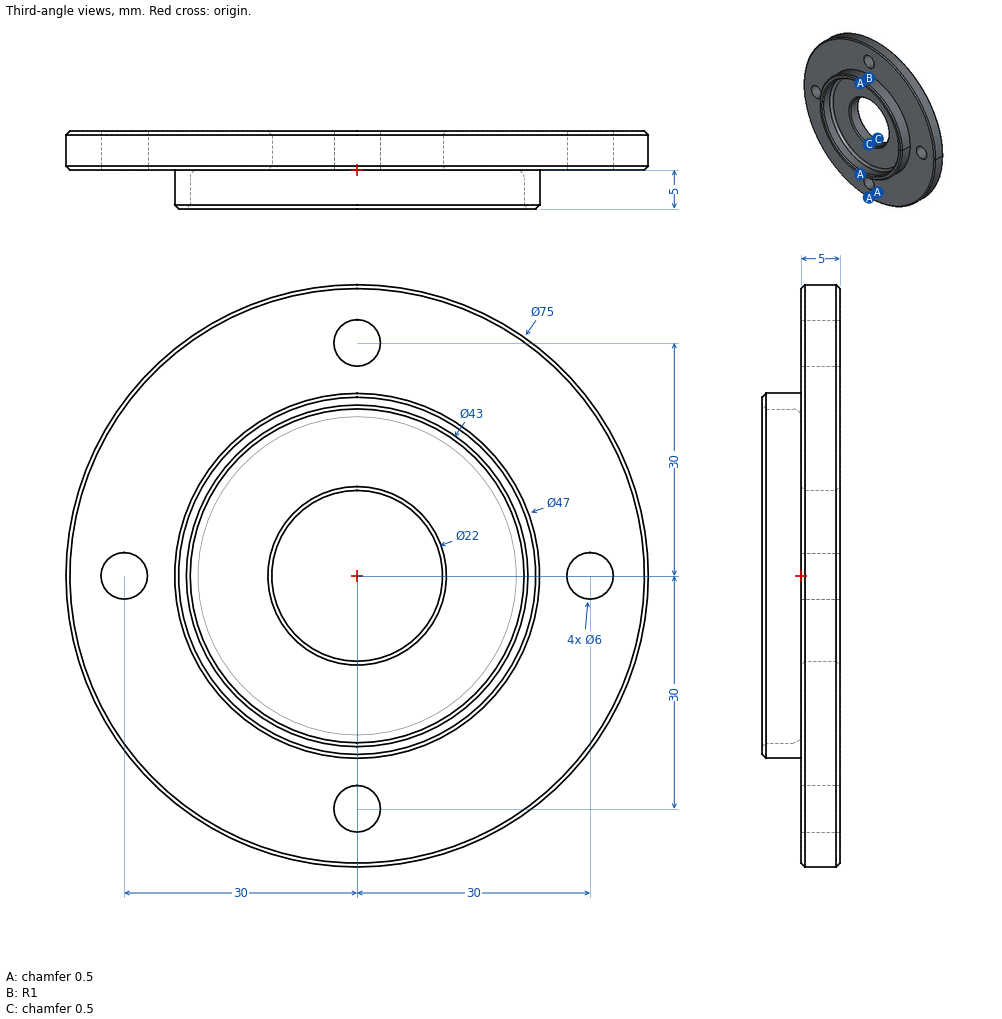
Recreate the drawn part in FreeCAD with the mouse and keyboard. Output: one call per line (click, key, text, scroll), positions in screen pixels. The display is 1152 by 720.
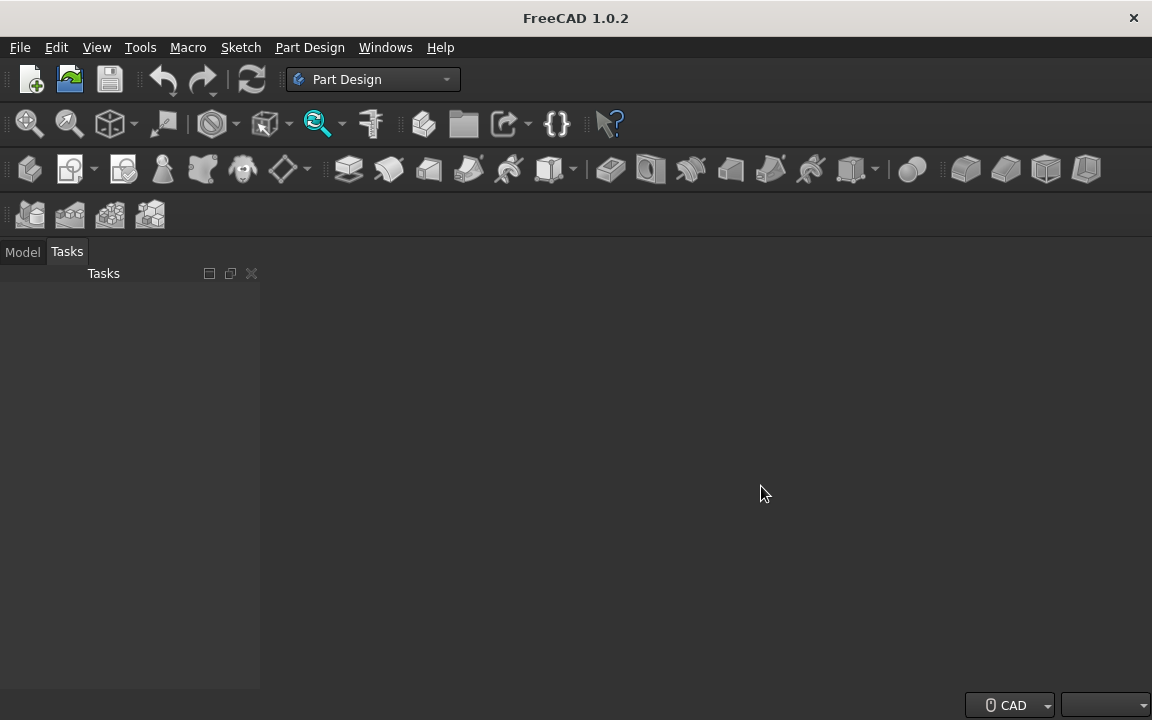
click(30, 80)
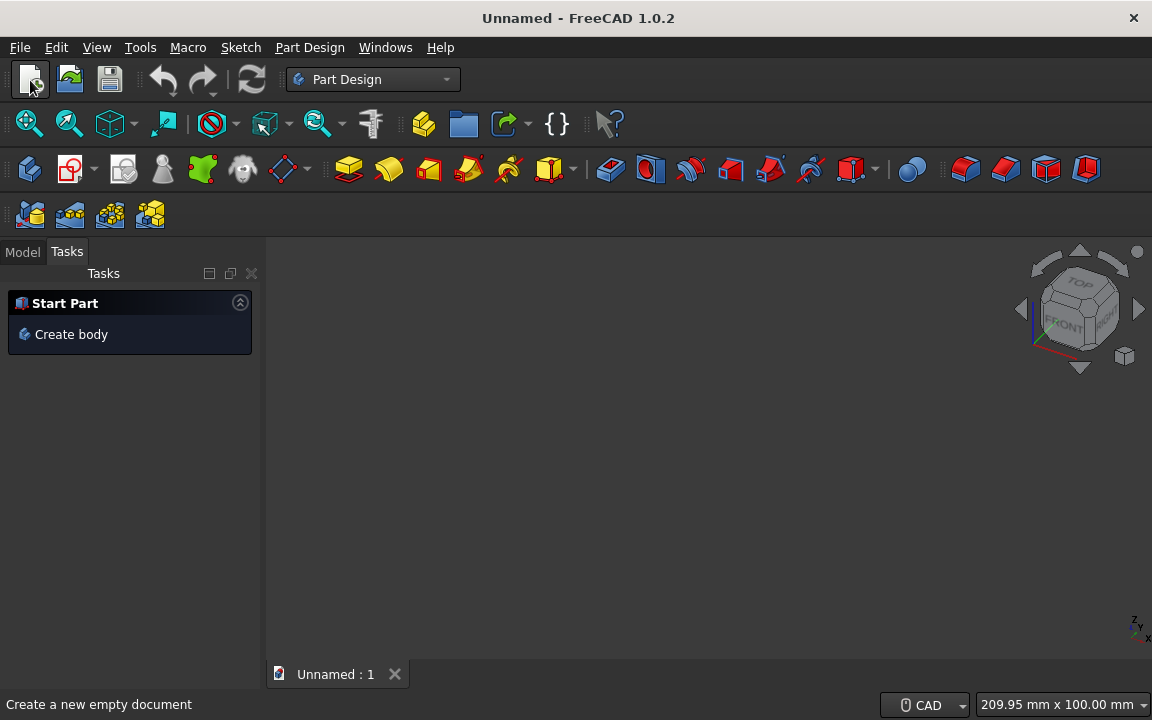
click(70, 170)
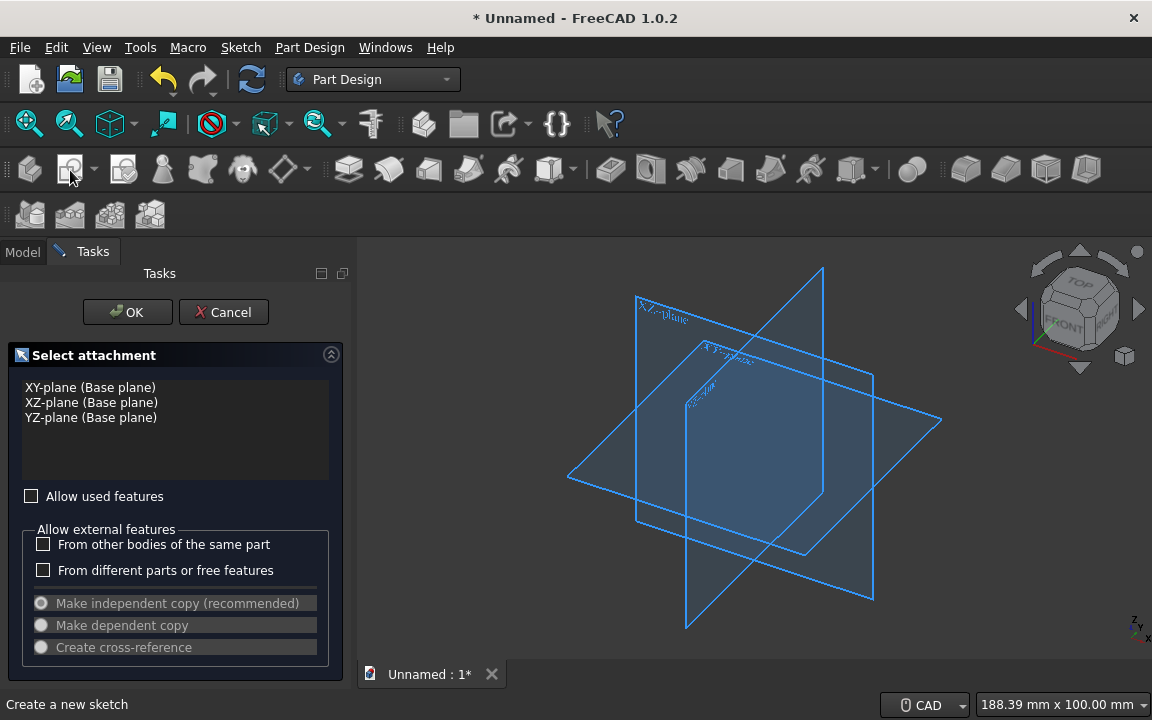
click(82, 402)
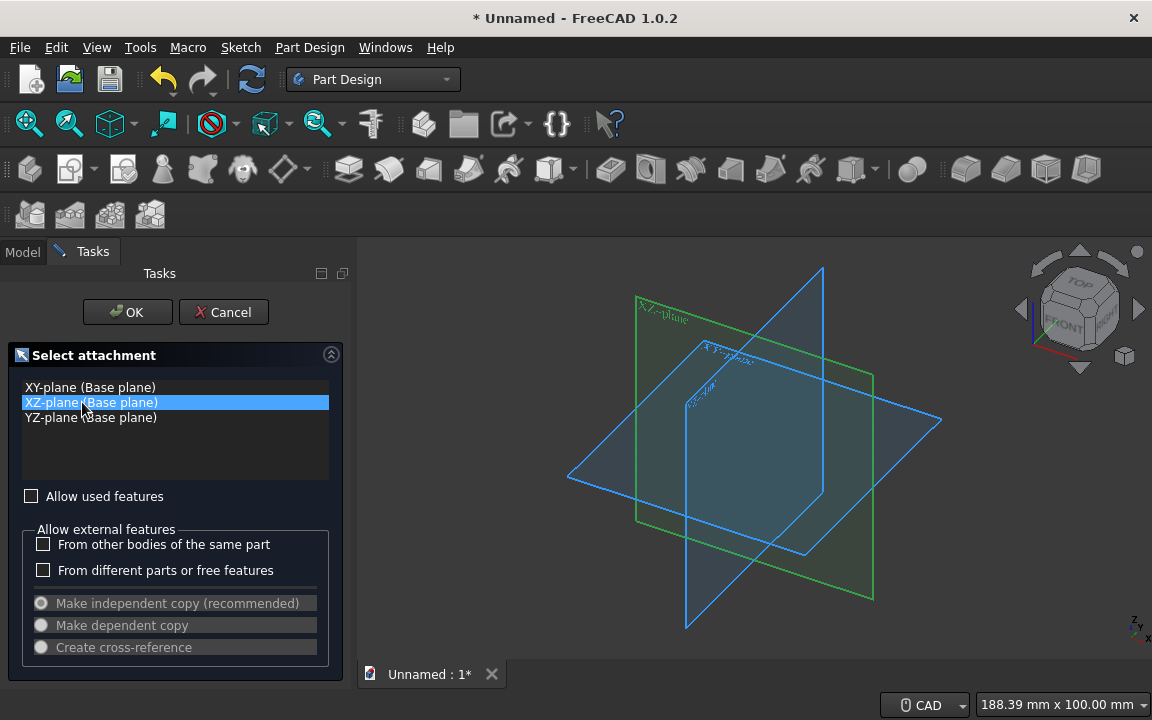
click(128, 312)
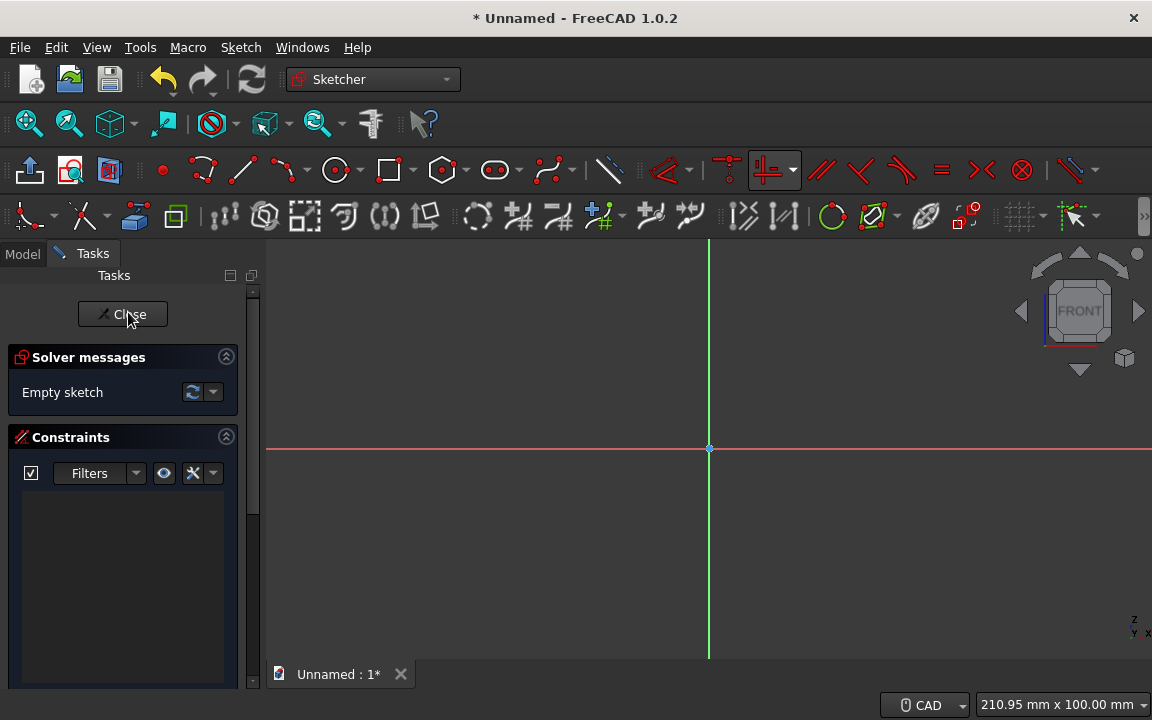
scroll(331, 449, down, 1)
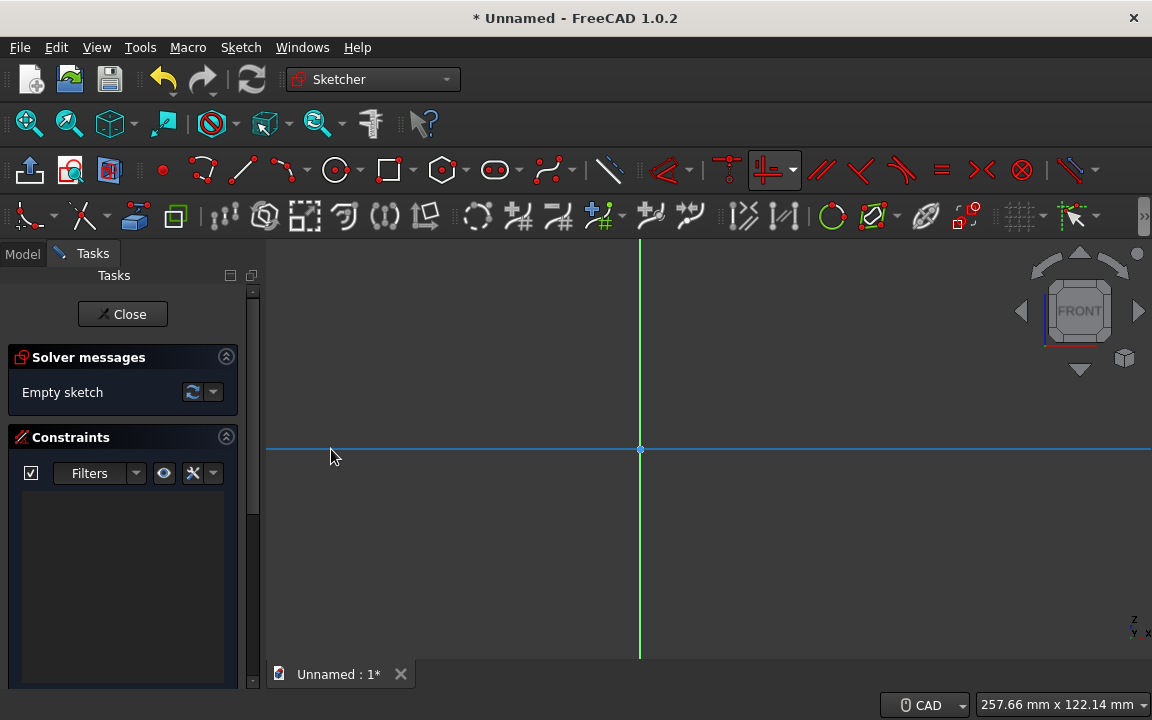
key(g)
key(c)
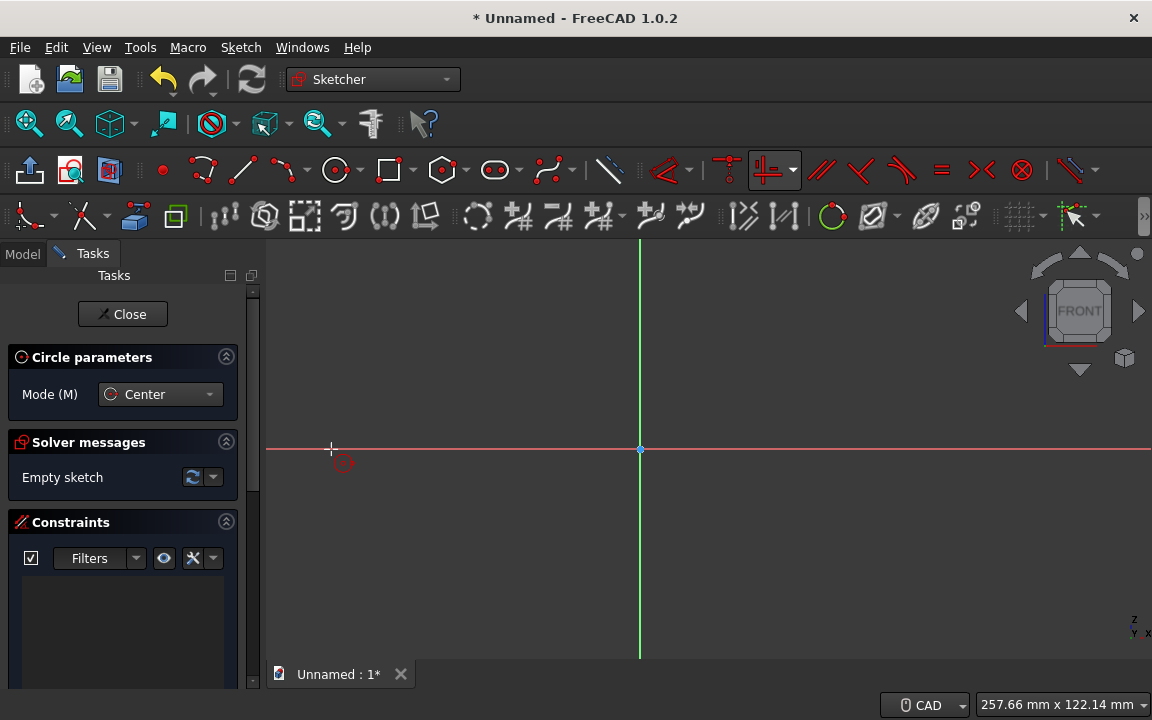
click(640, 449)
move(732, 358)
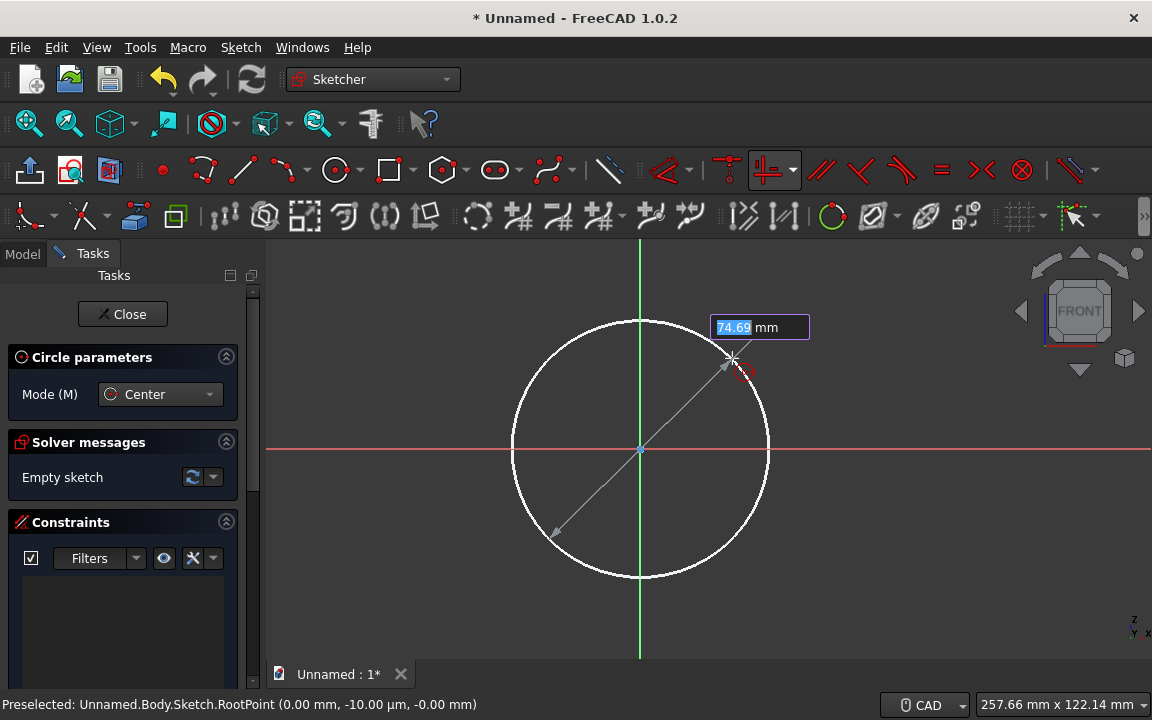
text(75)
key(Return)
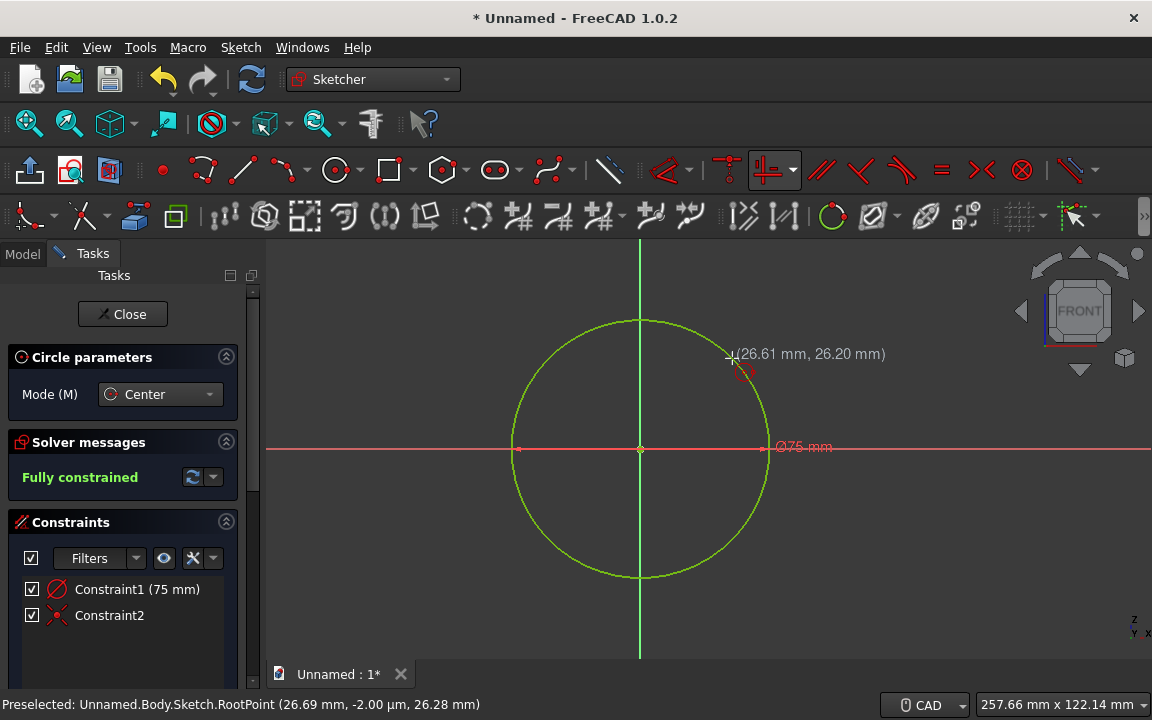
click(640, 449)
move(667, 422)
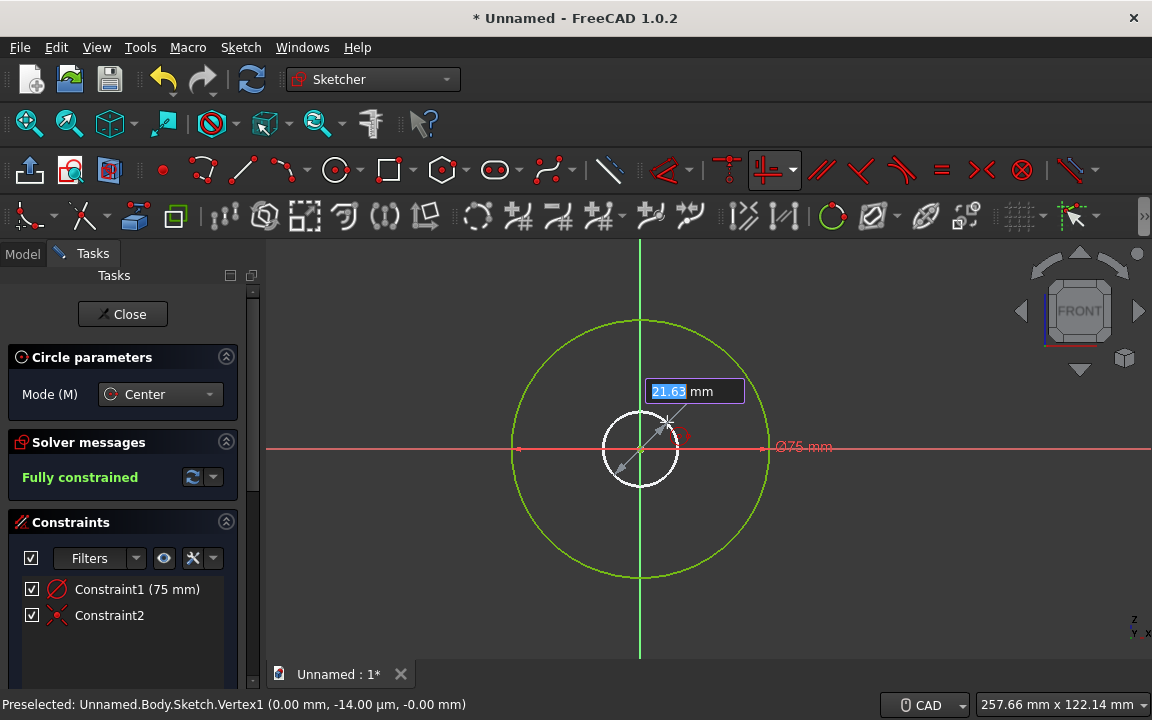
text(22)
key(Return)
key(Escape)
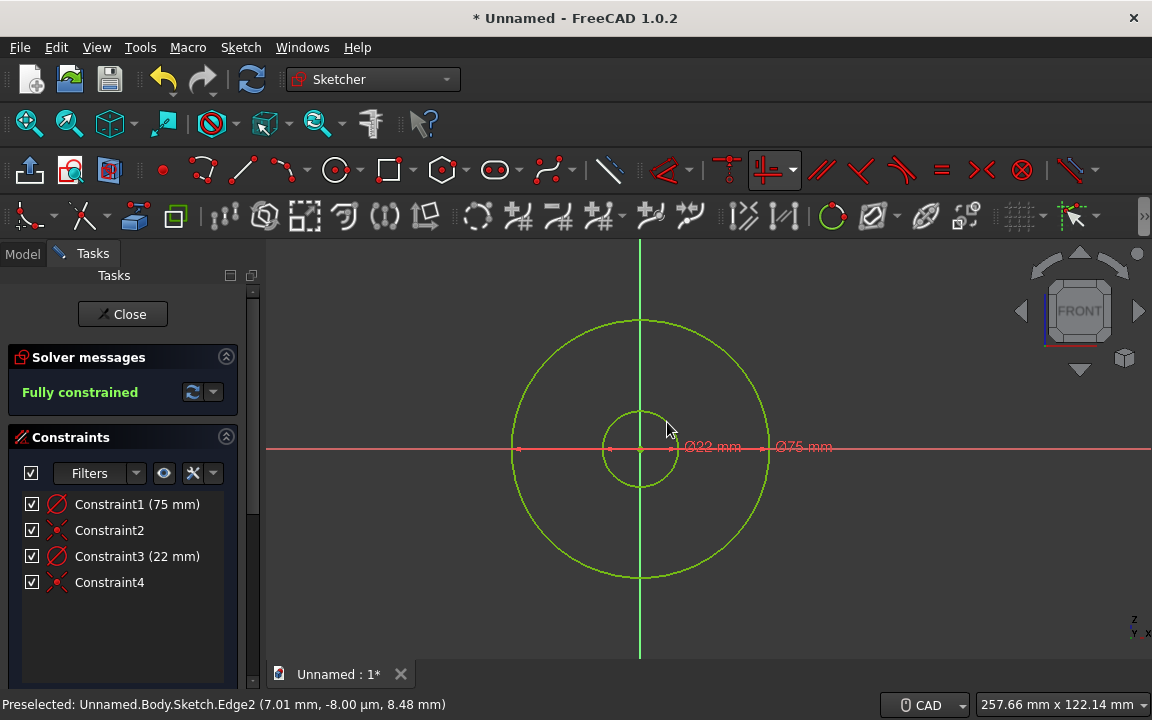
click(123, 314)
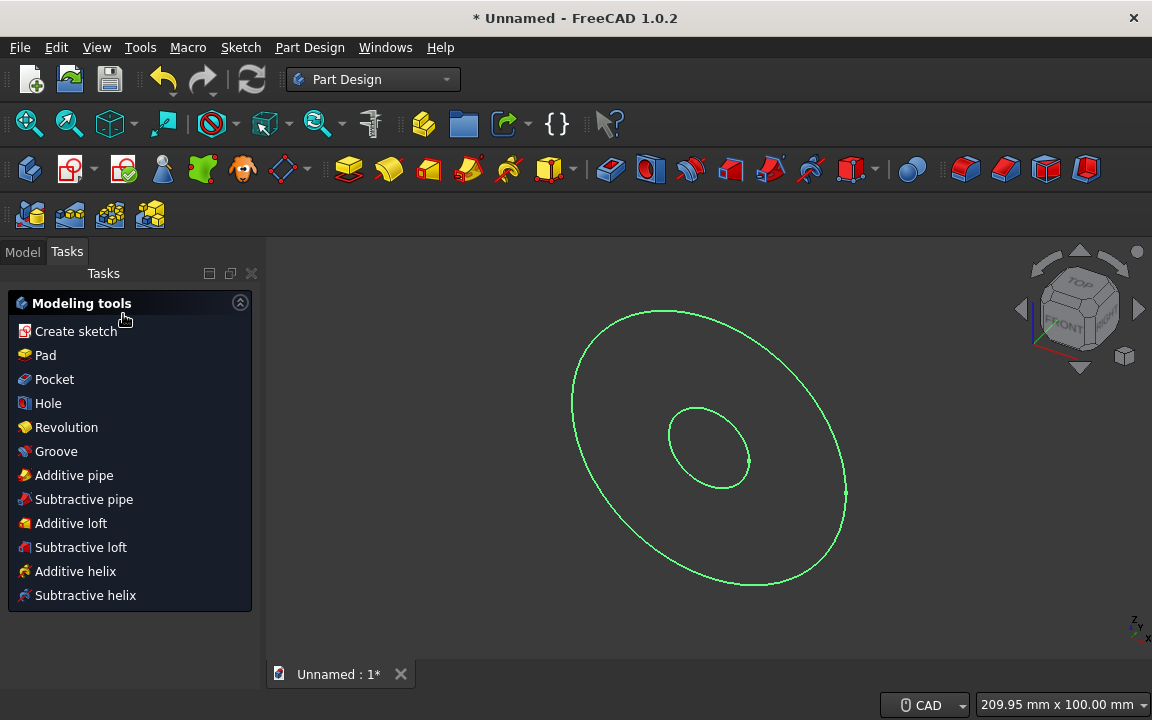
click(350, 170)